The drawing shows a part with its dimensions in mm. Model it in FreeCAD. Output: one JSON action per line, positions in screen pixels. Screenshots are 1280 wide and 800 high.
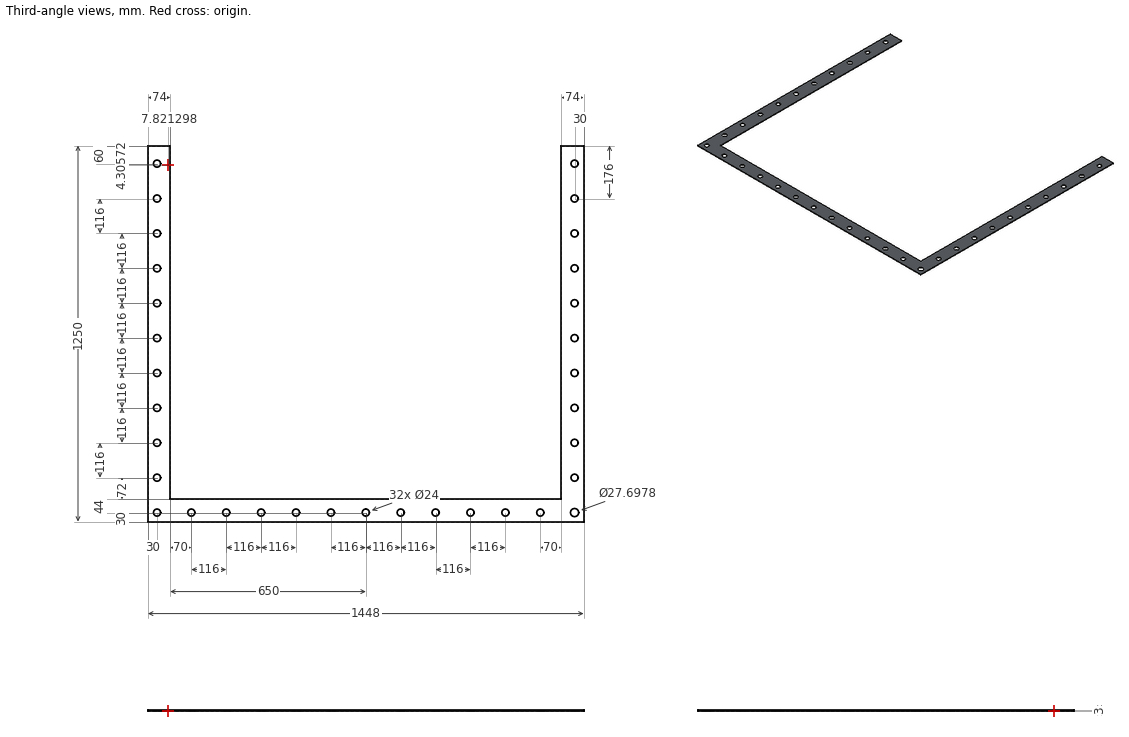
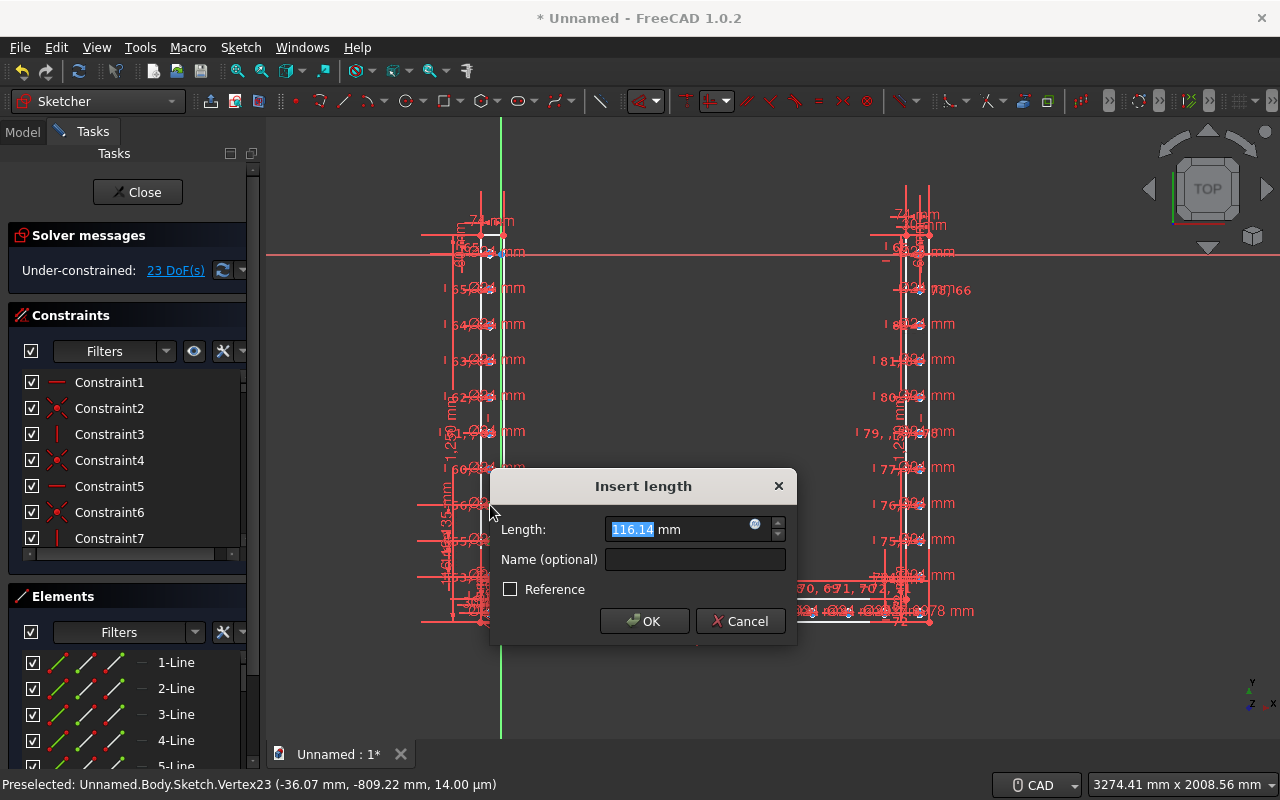
{"action": "type", "text": "116"}
{"action": "key", "text": "Return"}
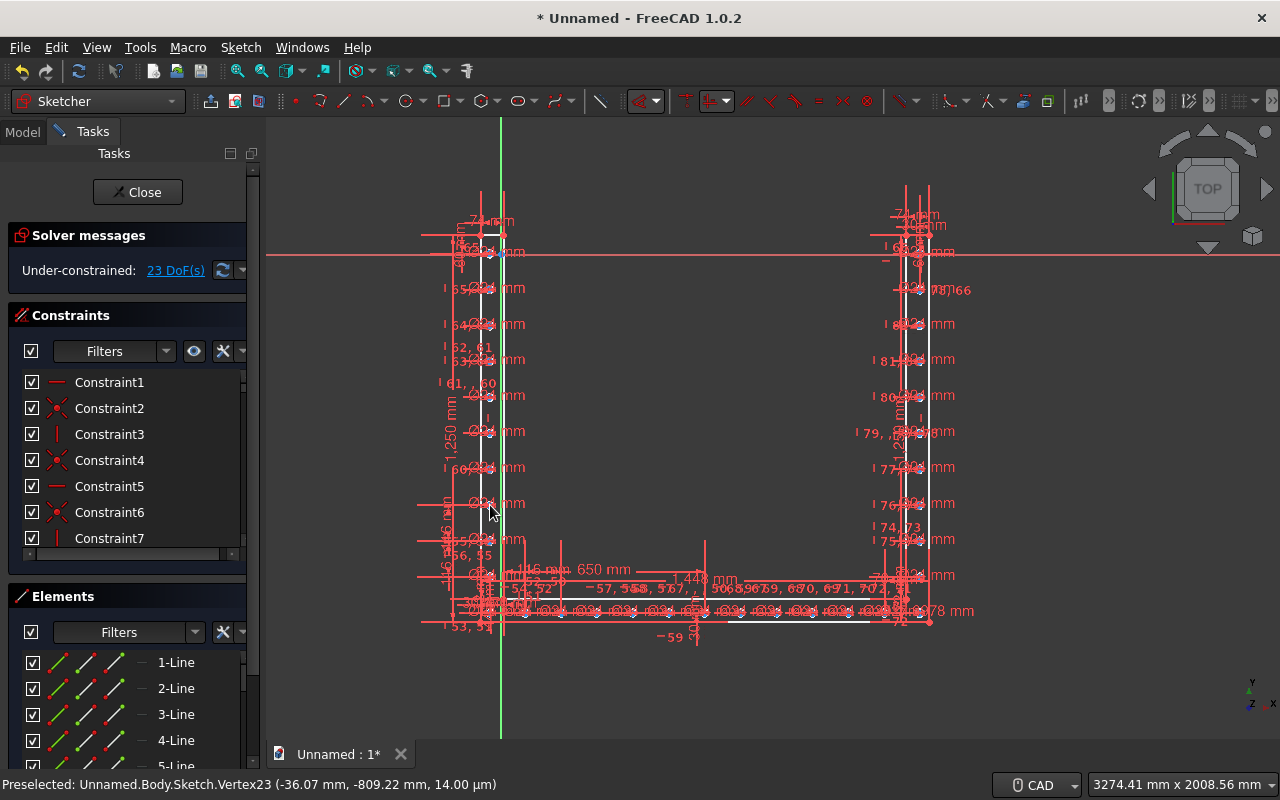
{"action": "left_click", "coordinate": [490, 505]}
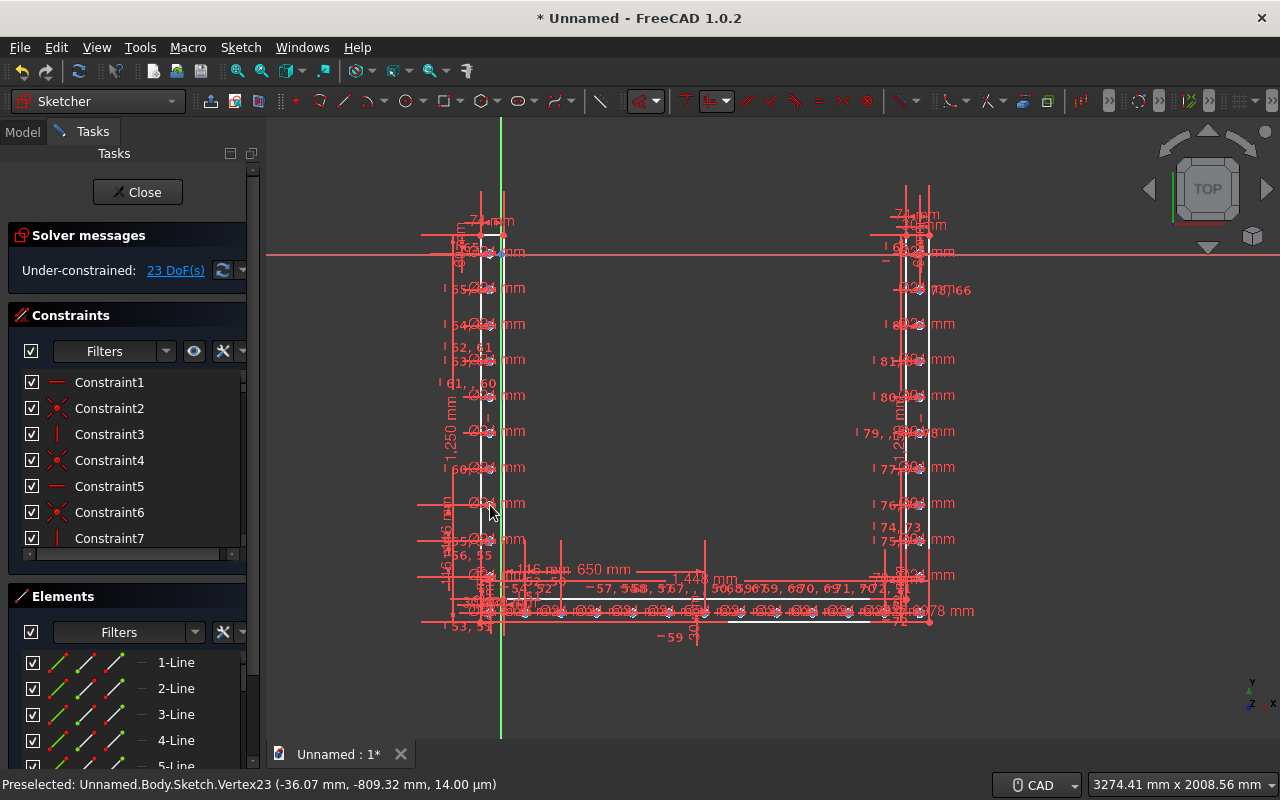
{"action": "left_click", "coordinate": [490, 469]}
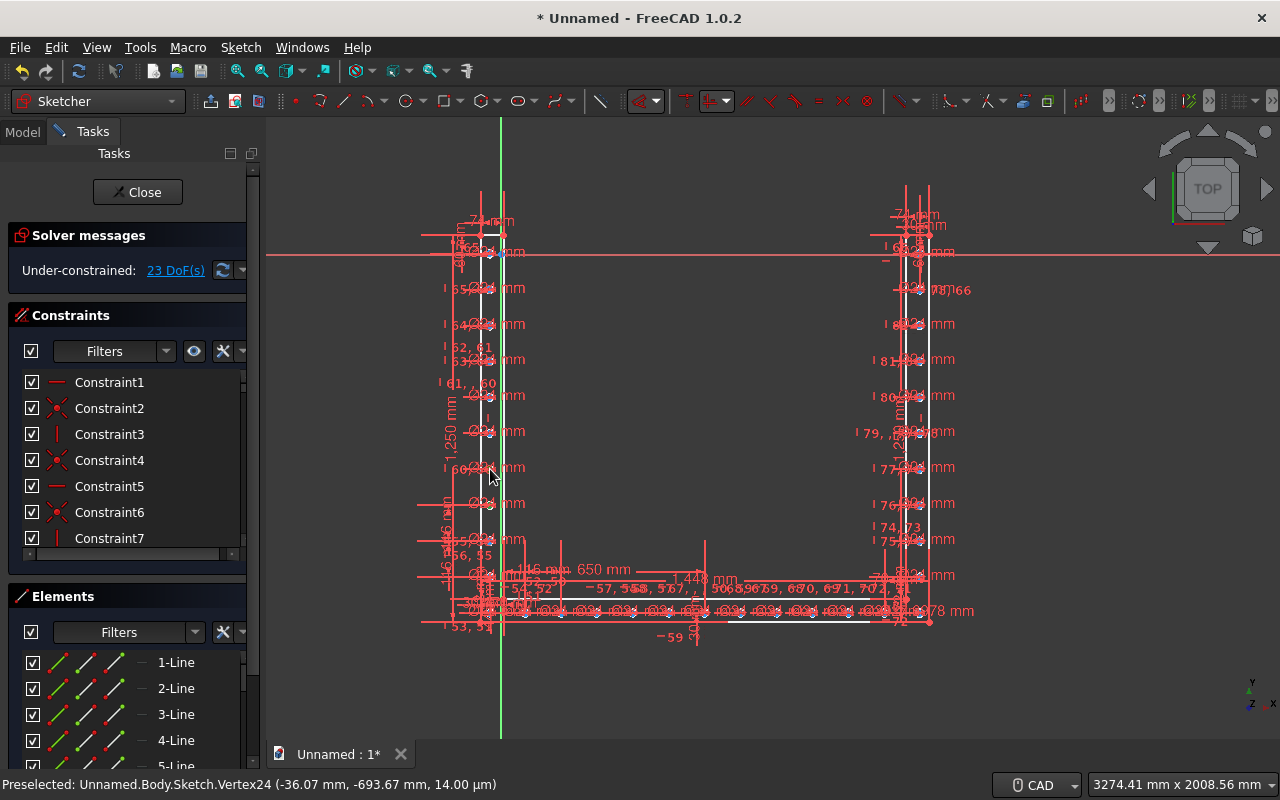
{"action": "key", "text": "i"}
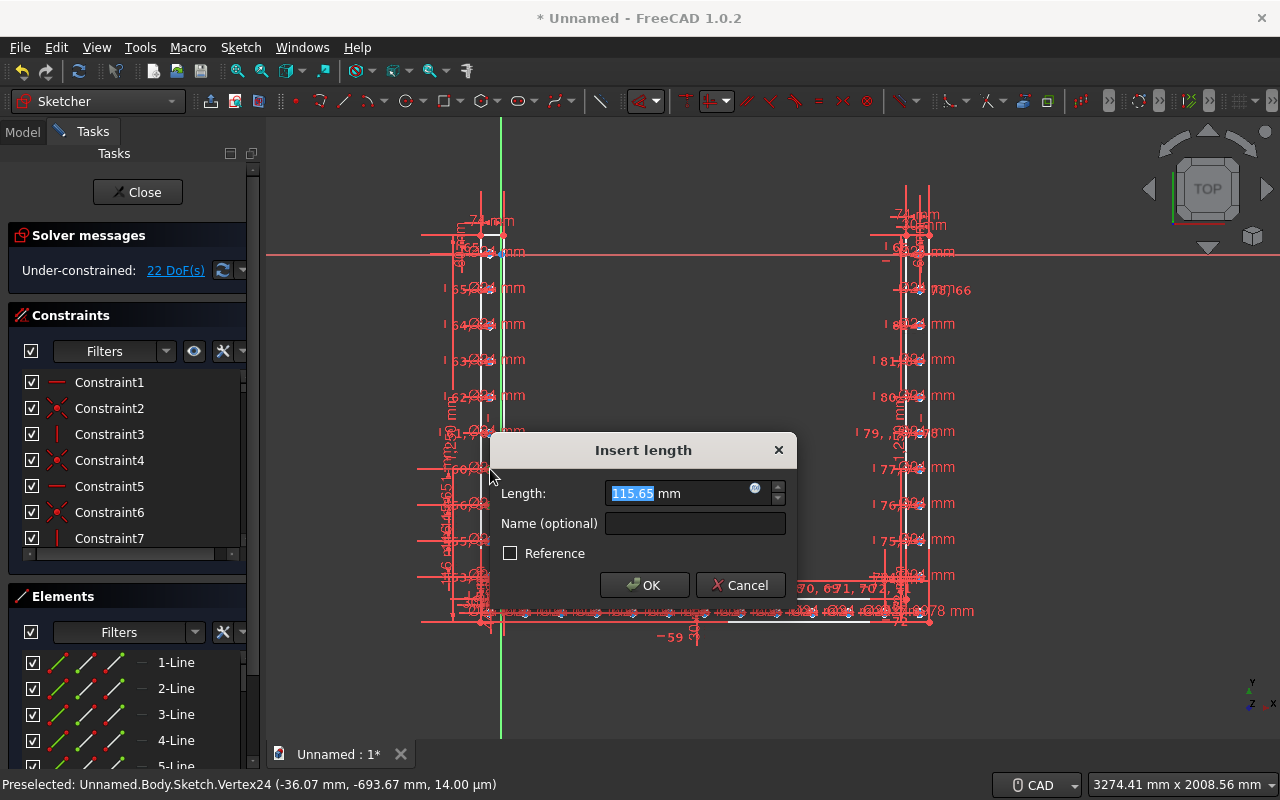
{"action": "type", "text": "116"}
{"action": "key", "text": "Return"}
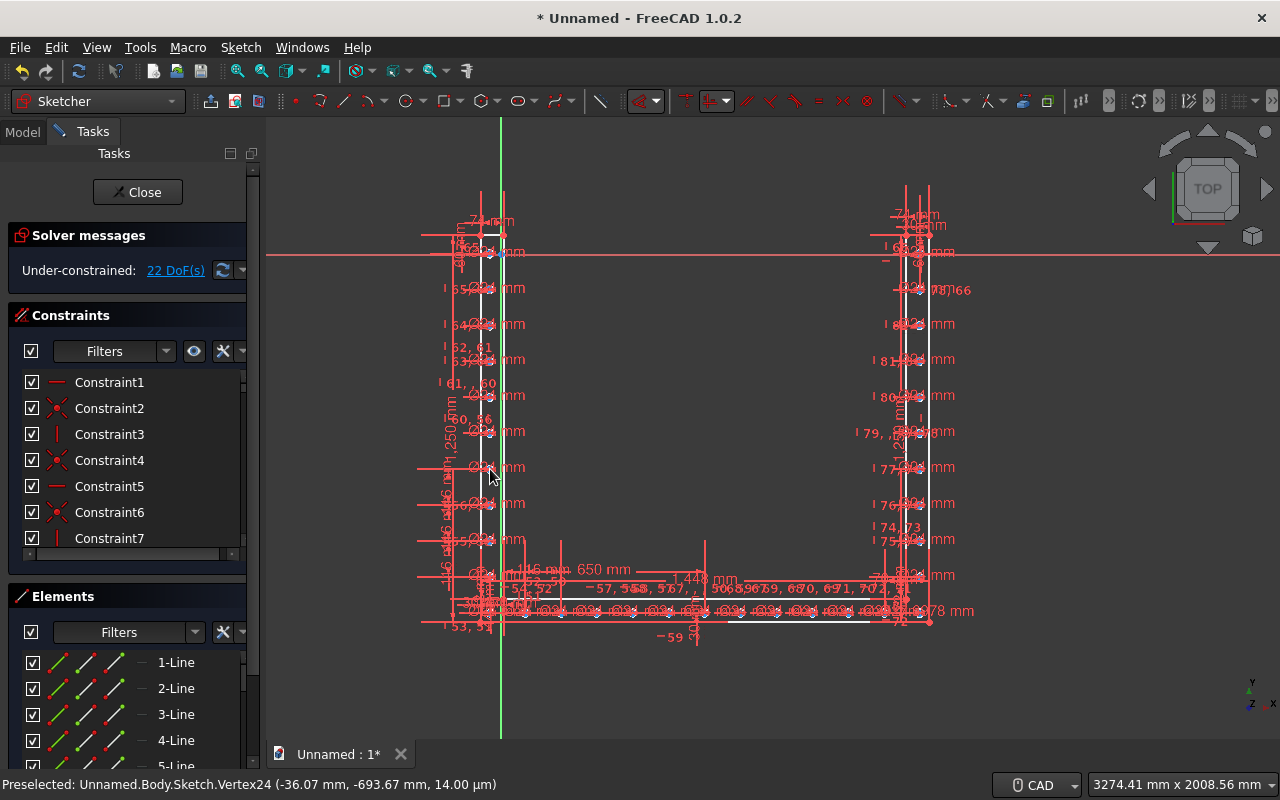
{"action": "left_click", "coordinate": [561, 613]}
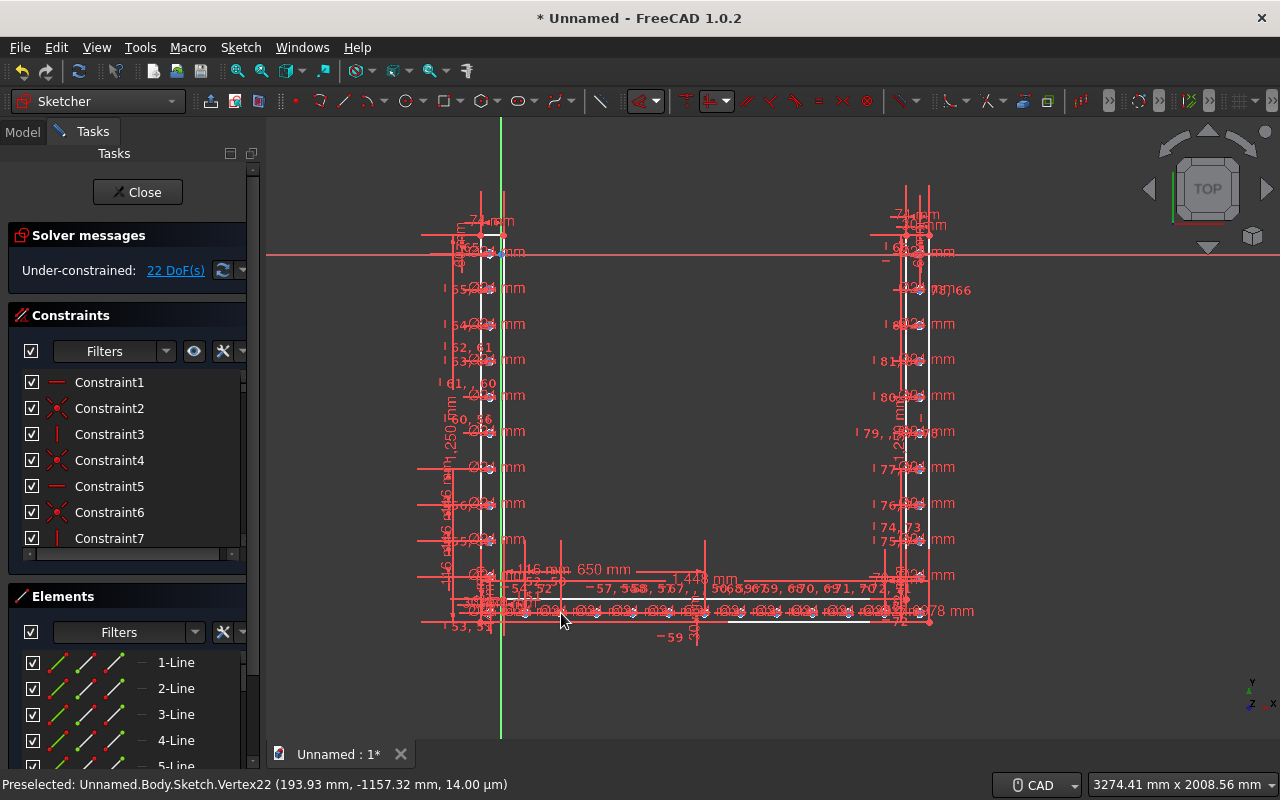
{"action": "left_click", "coordinate": [597, 613]}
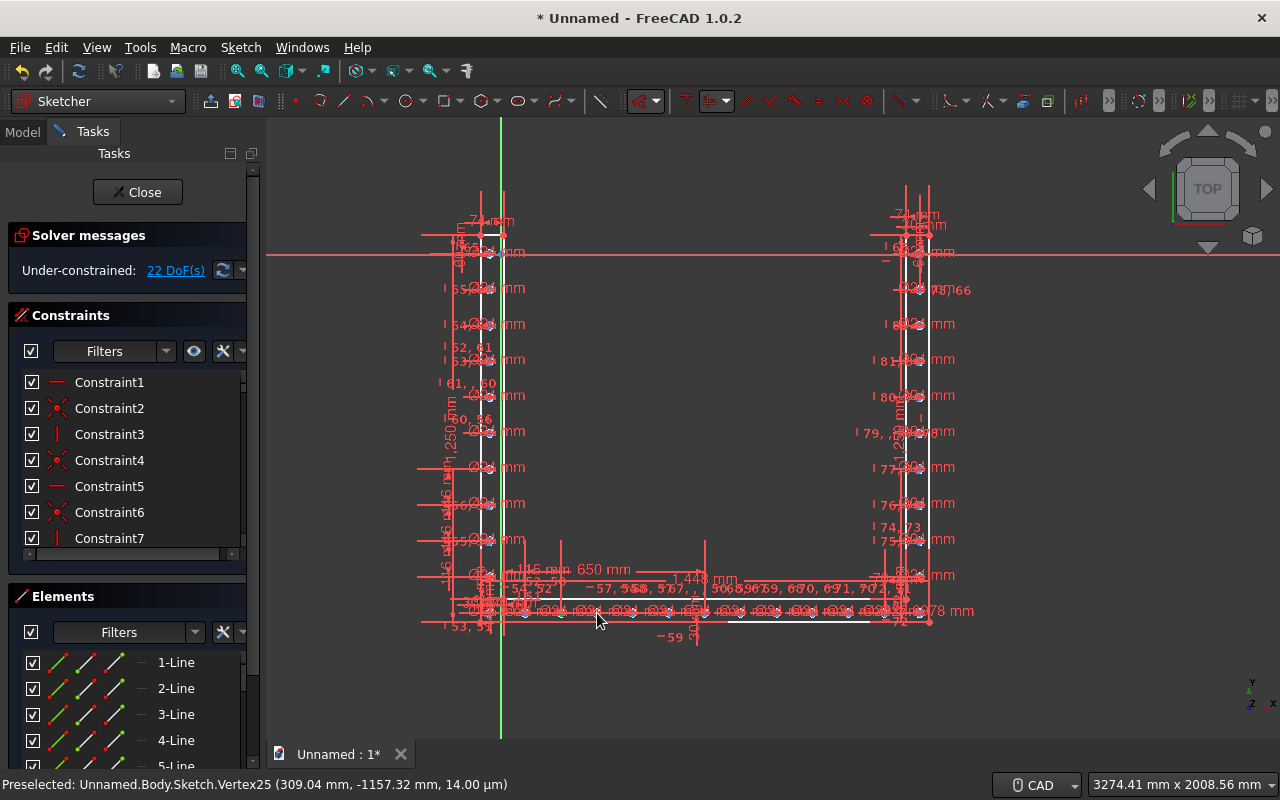
{"action": "key", "text": "l"}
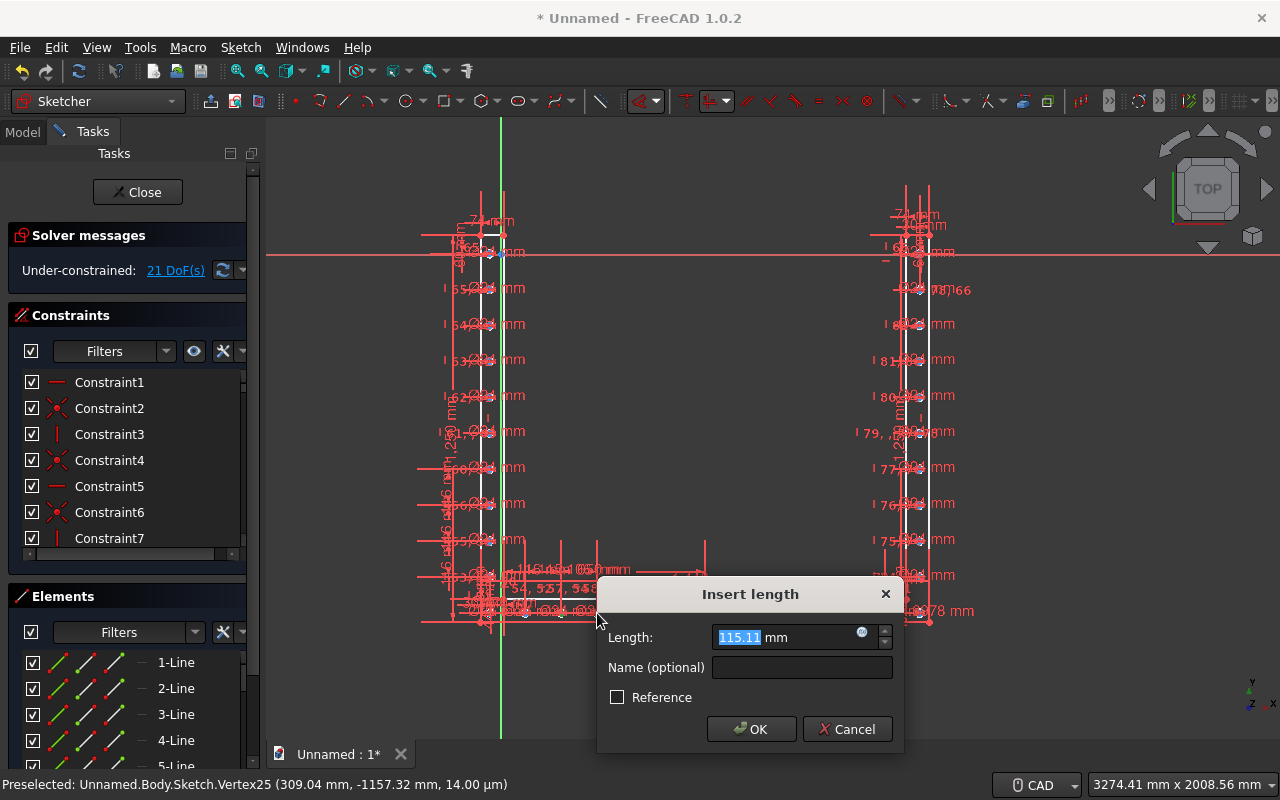
{"action": "type", "text": "116"}
{"action": "key", "text": "Return"}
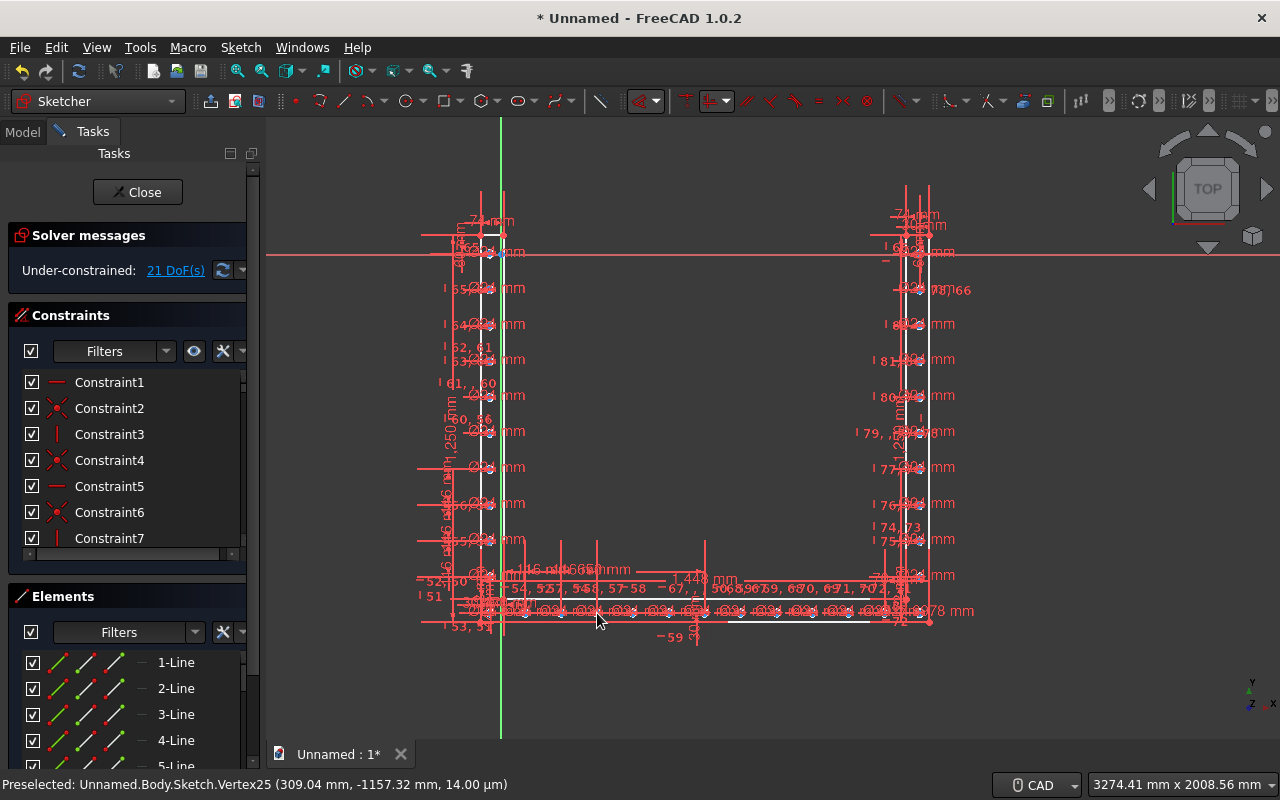
{"action": "left_click", "coordinate": [597, 613]}